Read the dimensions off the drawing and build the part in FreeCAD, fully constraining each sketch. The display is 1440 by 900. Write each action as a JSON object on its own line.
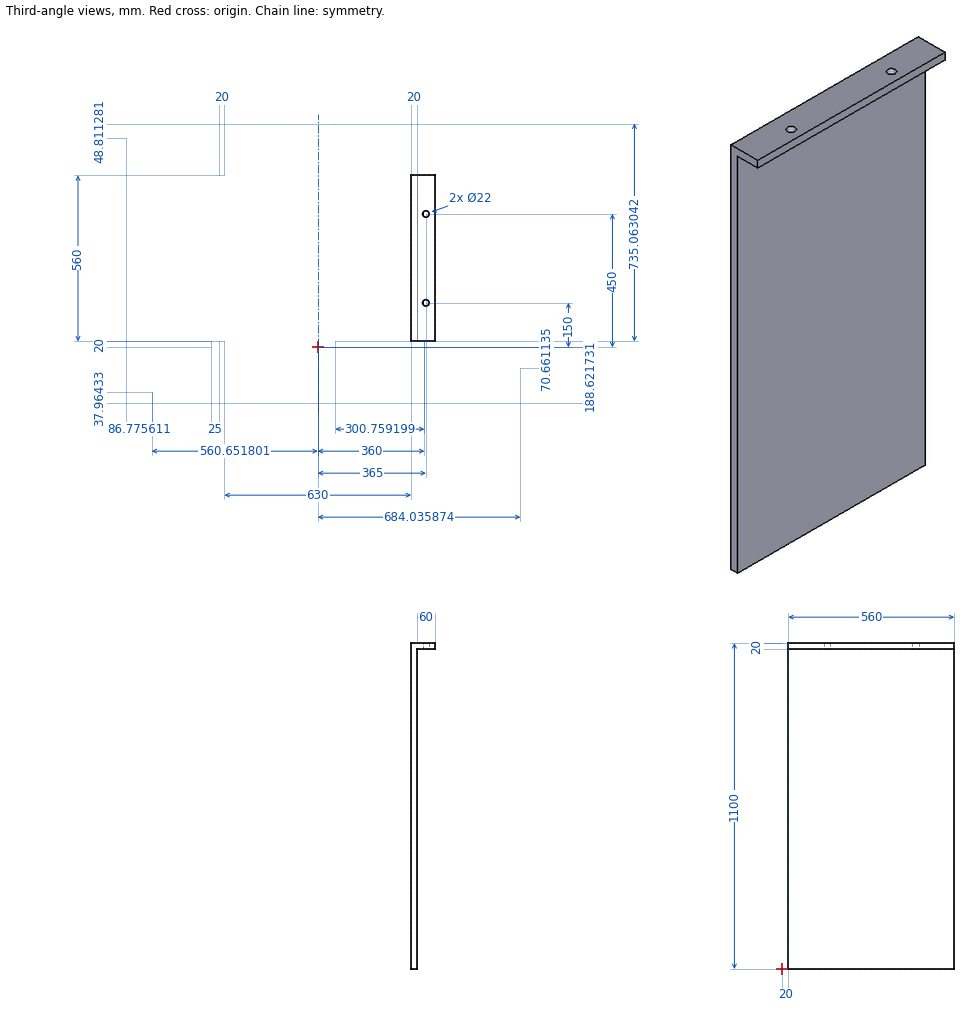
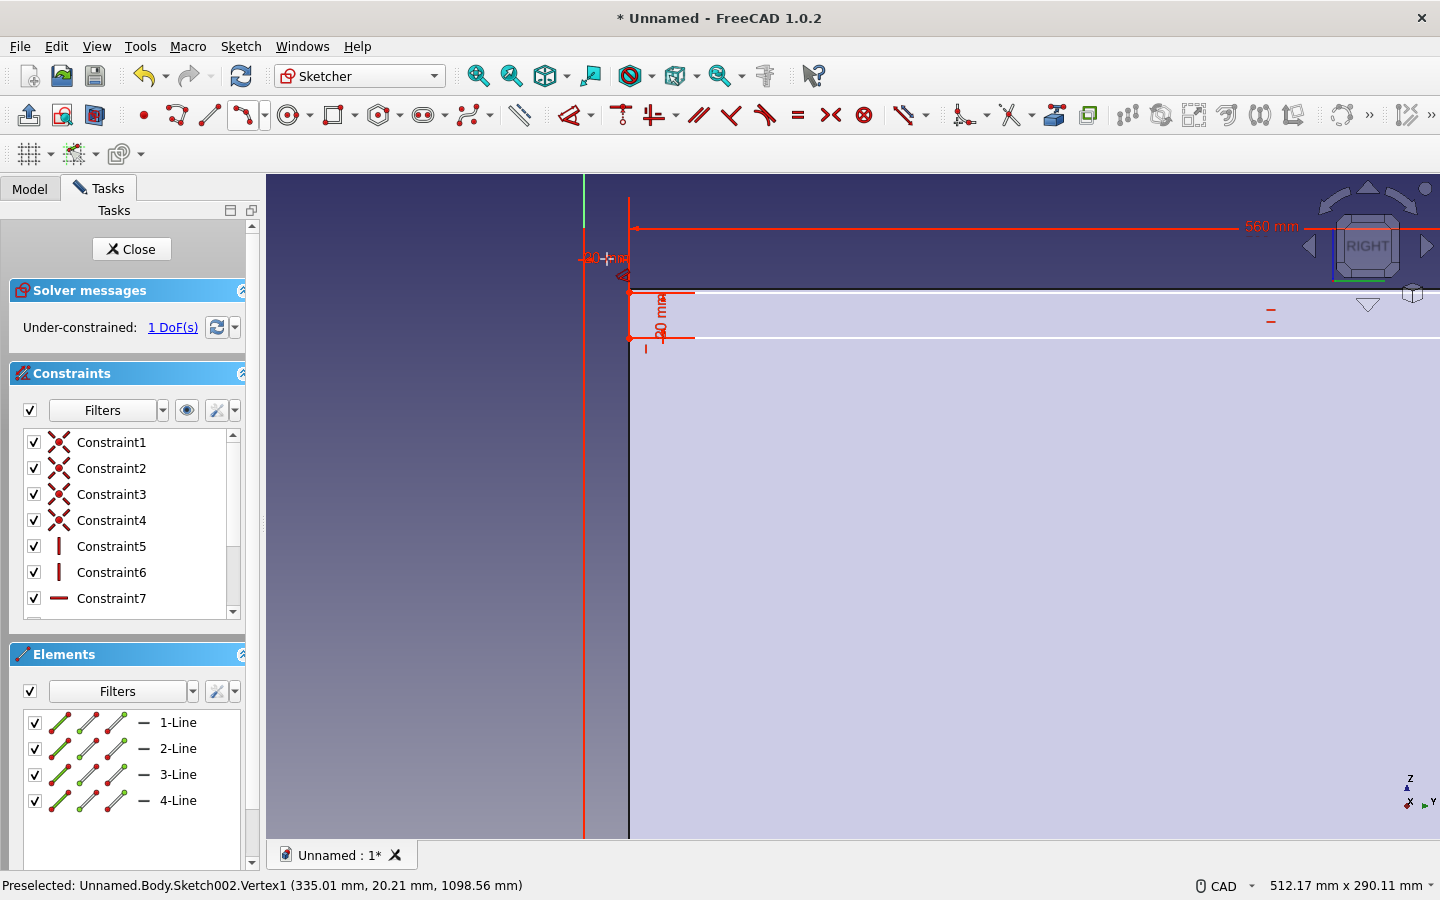
{"action": "scroll", "coordinate": [693, 300], "scroll_direction": "down", "scroll_amount": 9}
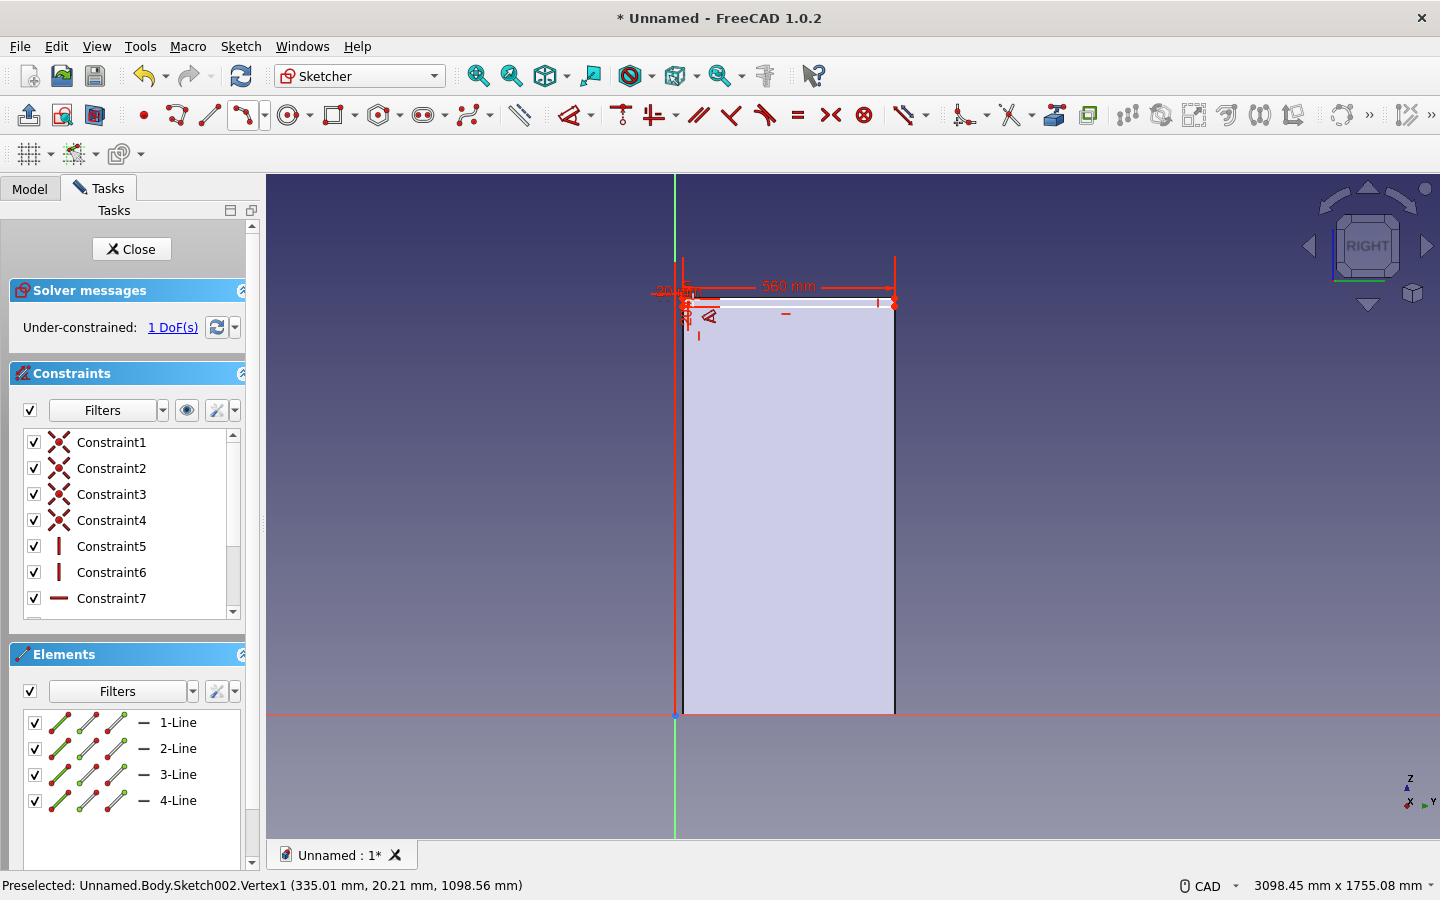
{"action": "scroll", "coordinate": [683, 299], "scroll_direction": "up", "scroll_amount": 3}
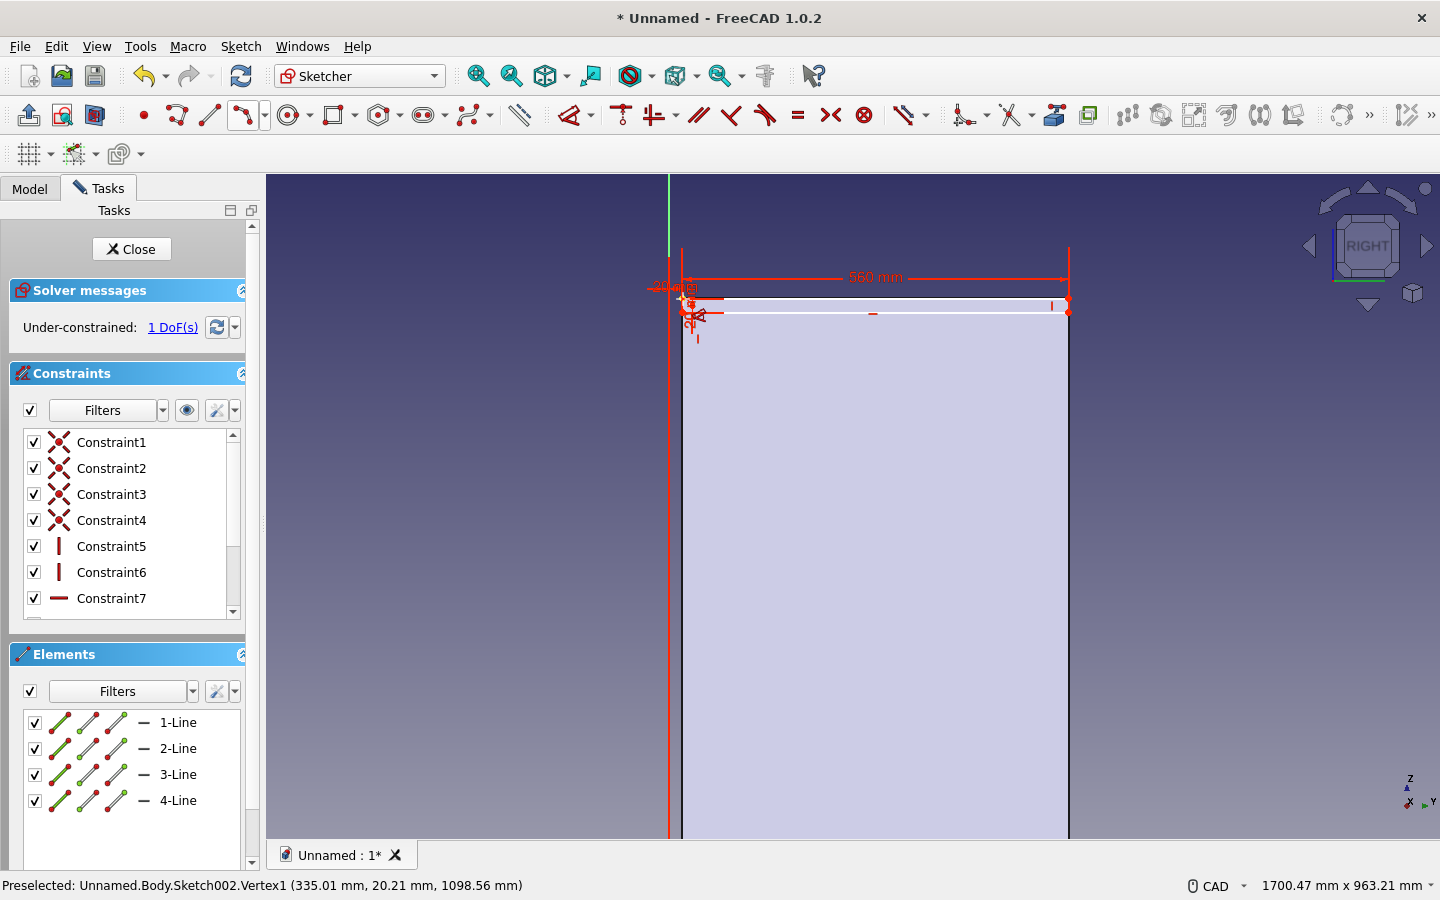
{"action": "left_click", "coordinate": [682, 299]}
{"action": "left_click", "coordinate": [635, 555]}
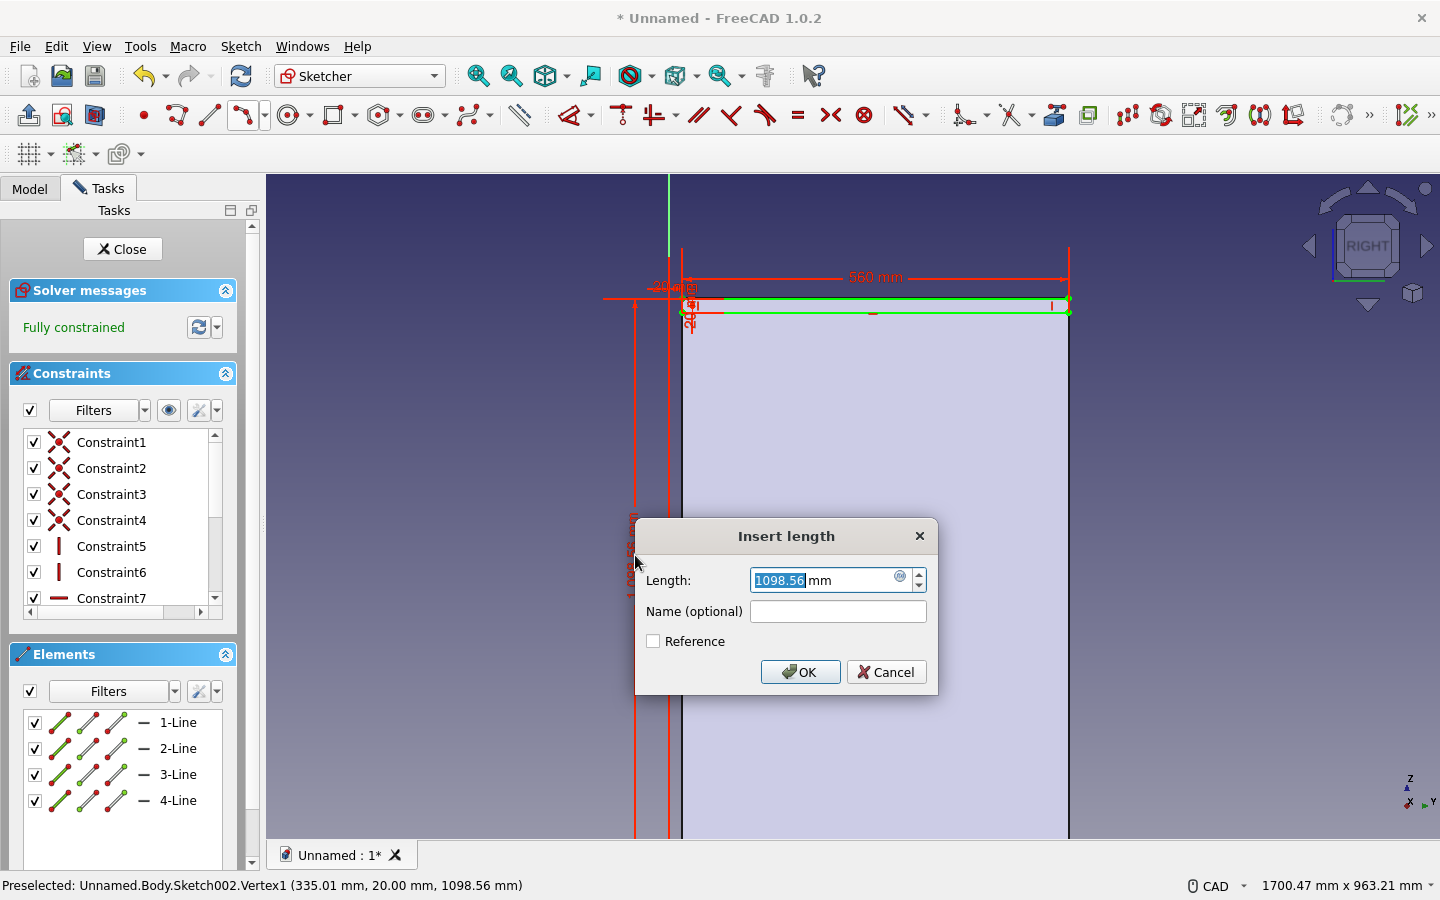
{"action": "type", "text": "1100"}
{"action": "key", "text": "Return"}
{"action": "key", "text": "Escape"}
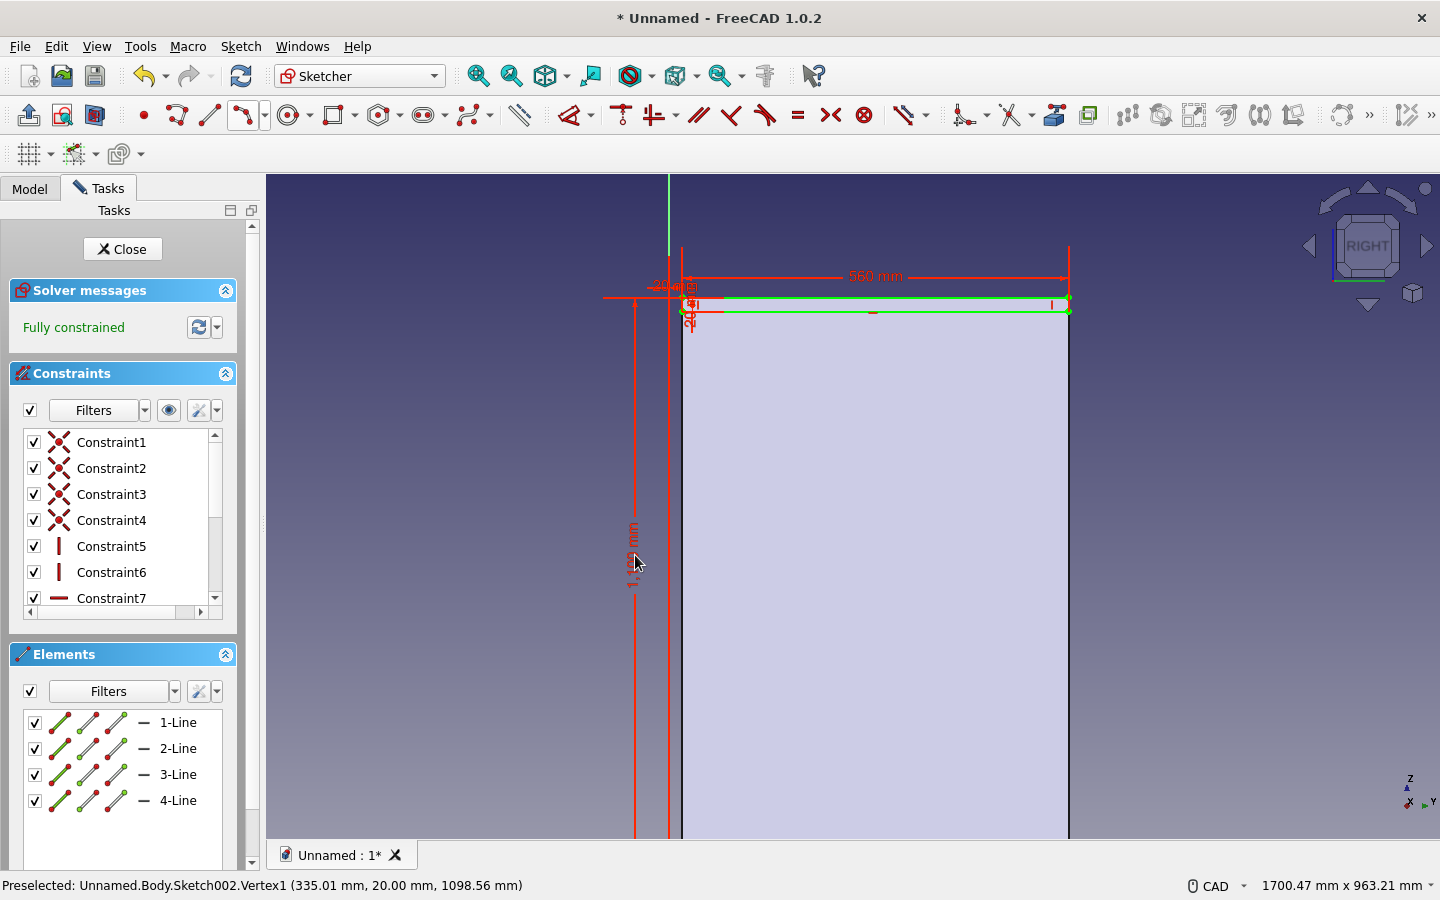
{"action": "left_click", "coordinate": [123, 249]}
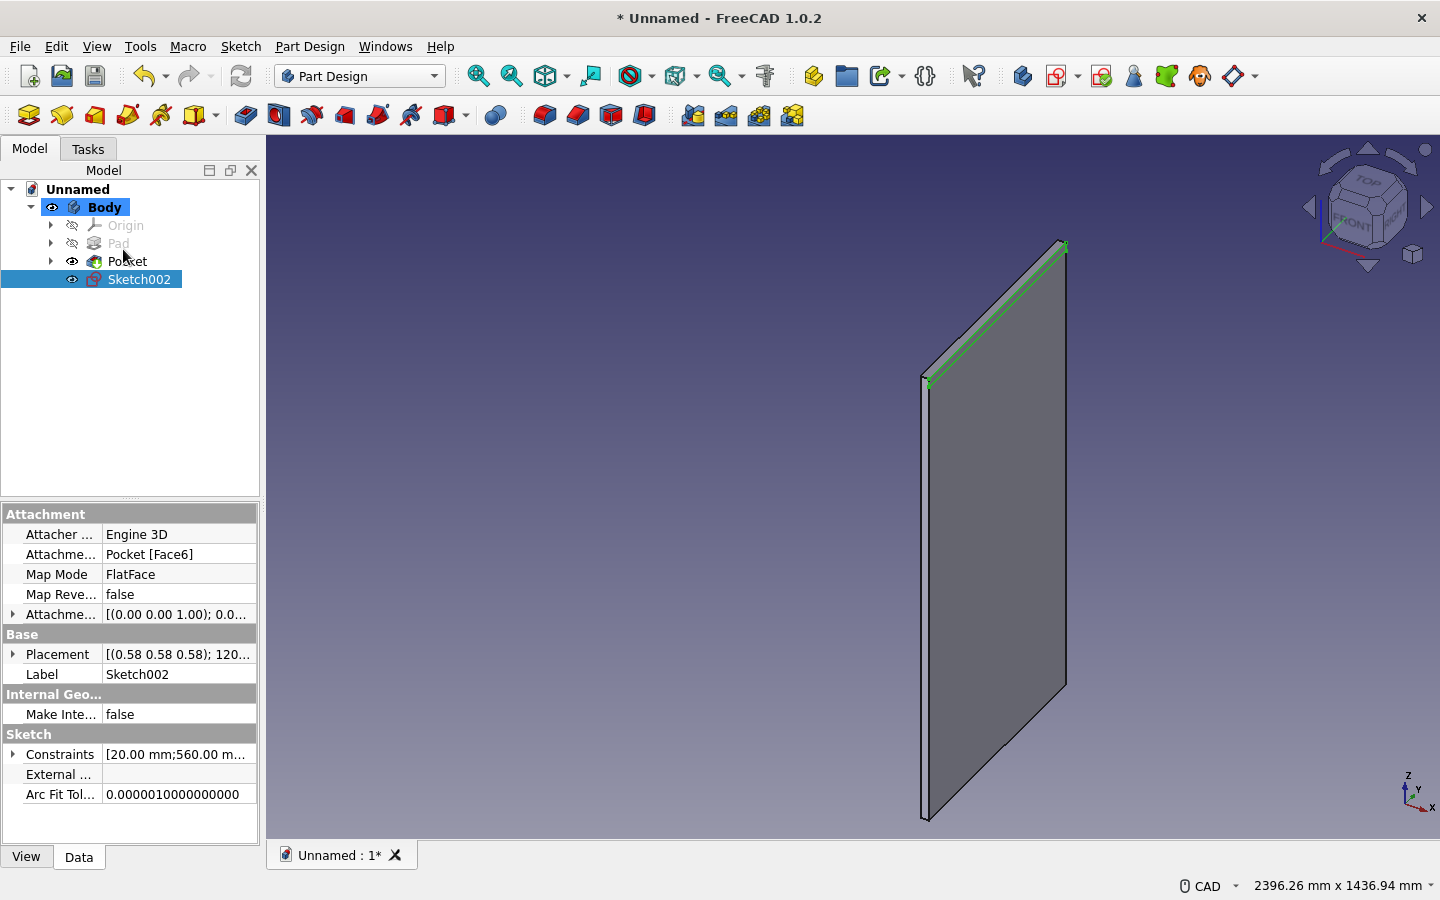
{"action": "left_click", "coordinate": [29, 116]}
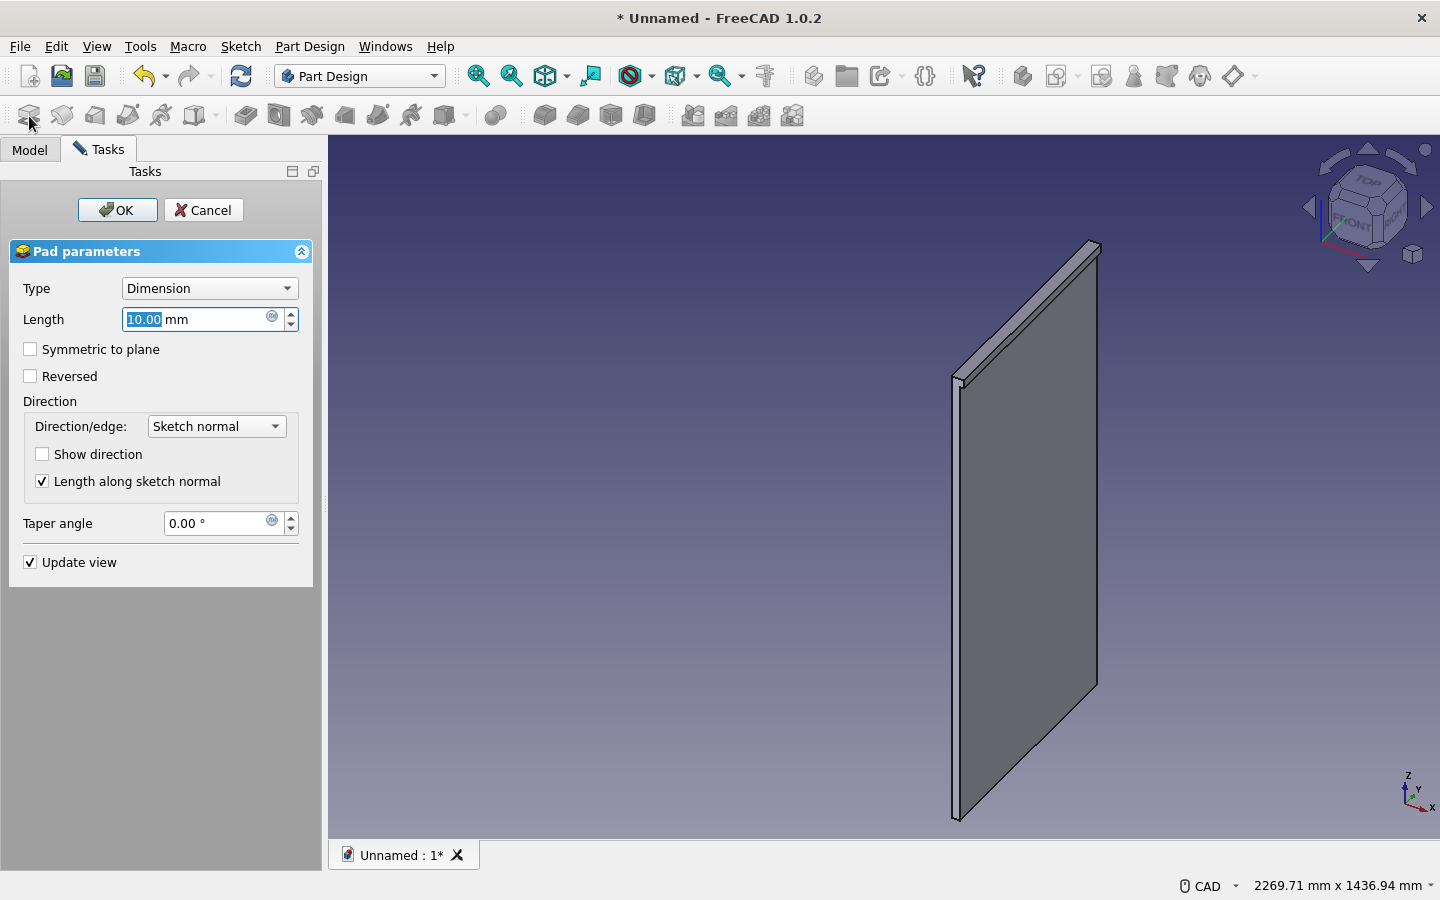
{"action": "type", "text": "60"}
{"action": "key", "text": "Tab"}